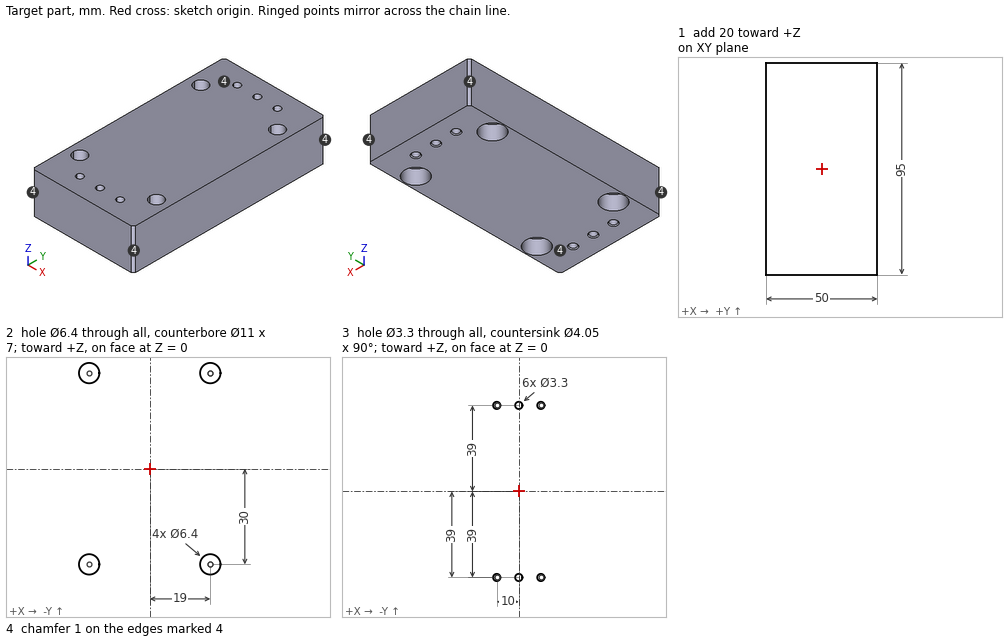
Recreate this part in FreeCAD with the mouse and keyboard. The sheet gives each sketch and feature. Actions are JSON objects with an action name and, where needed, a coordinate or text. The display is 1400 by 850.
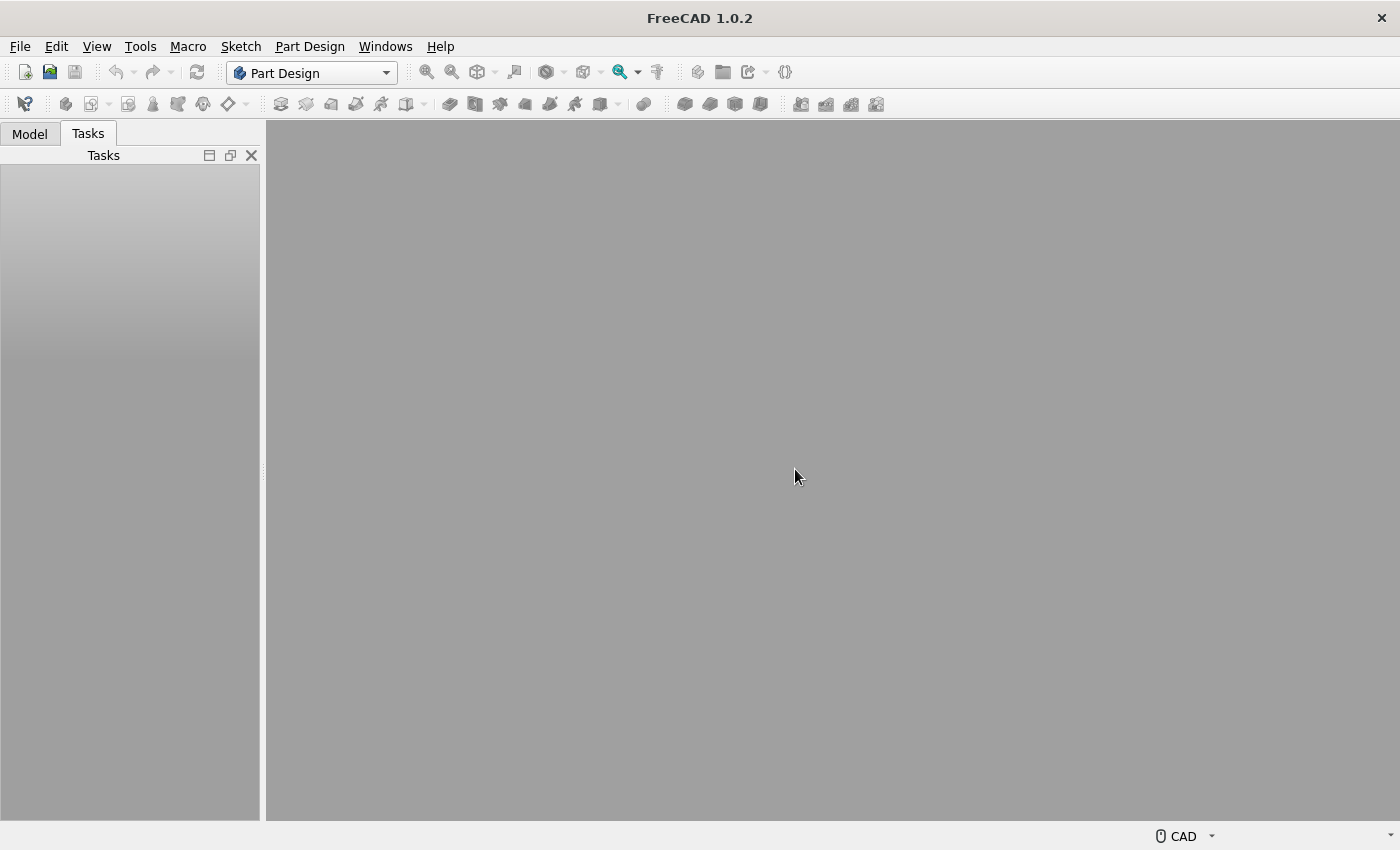
{"action": "left_click", "coordinate": [25, 72]}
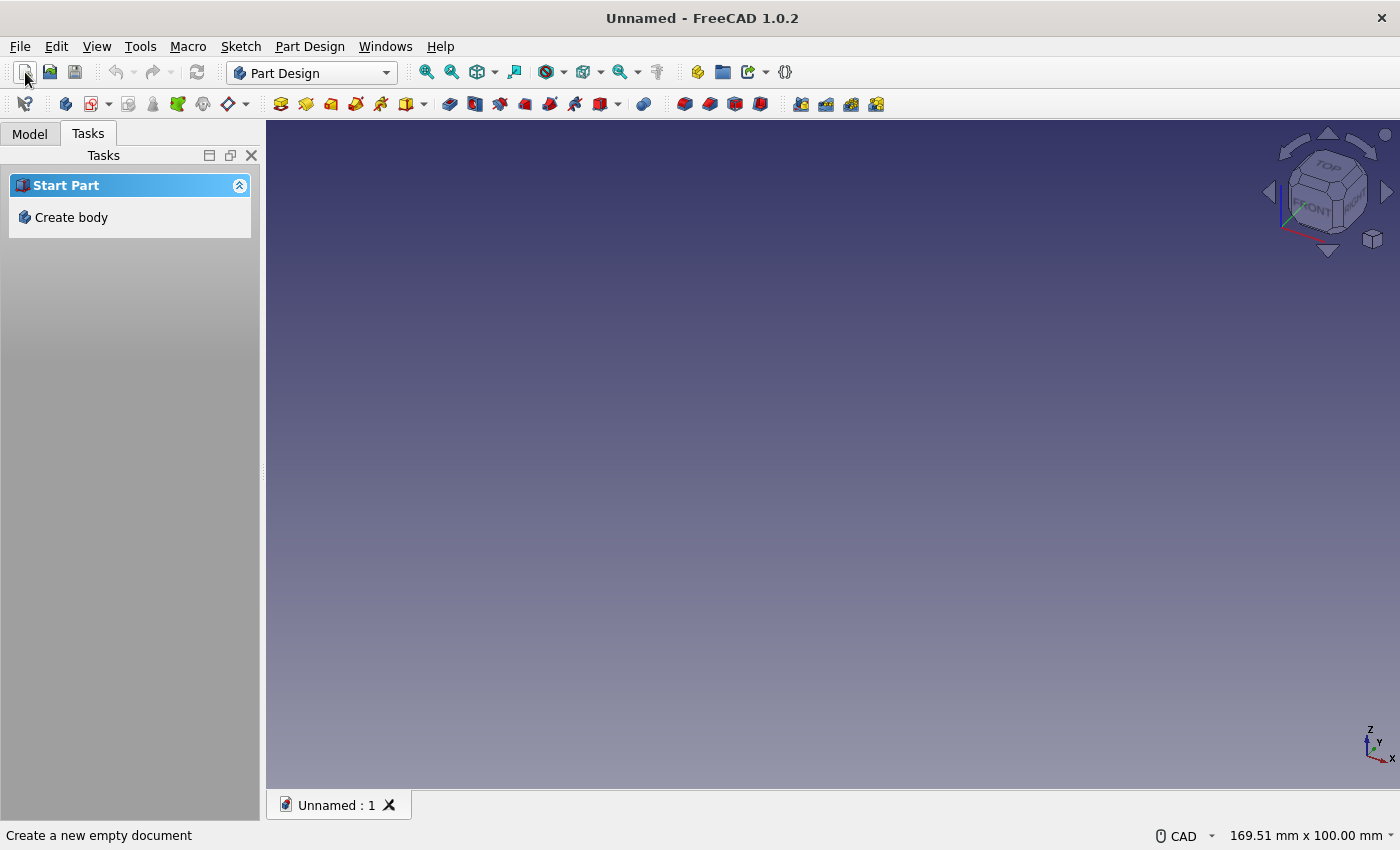
{"action": "left_click", "coordinate": [90, 104]}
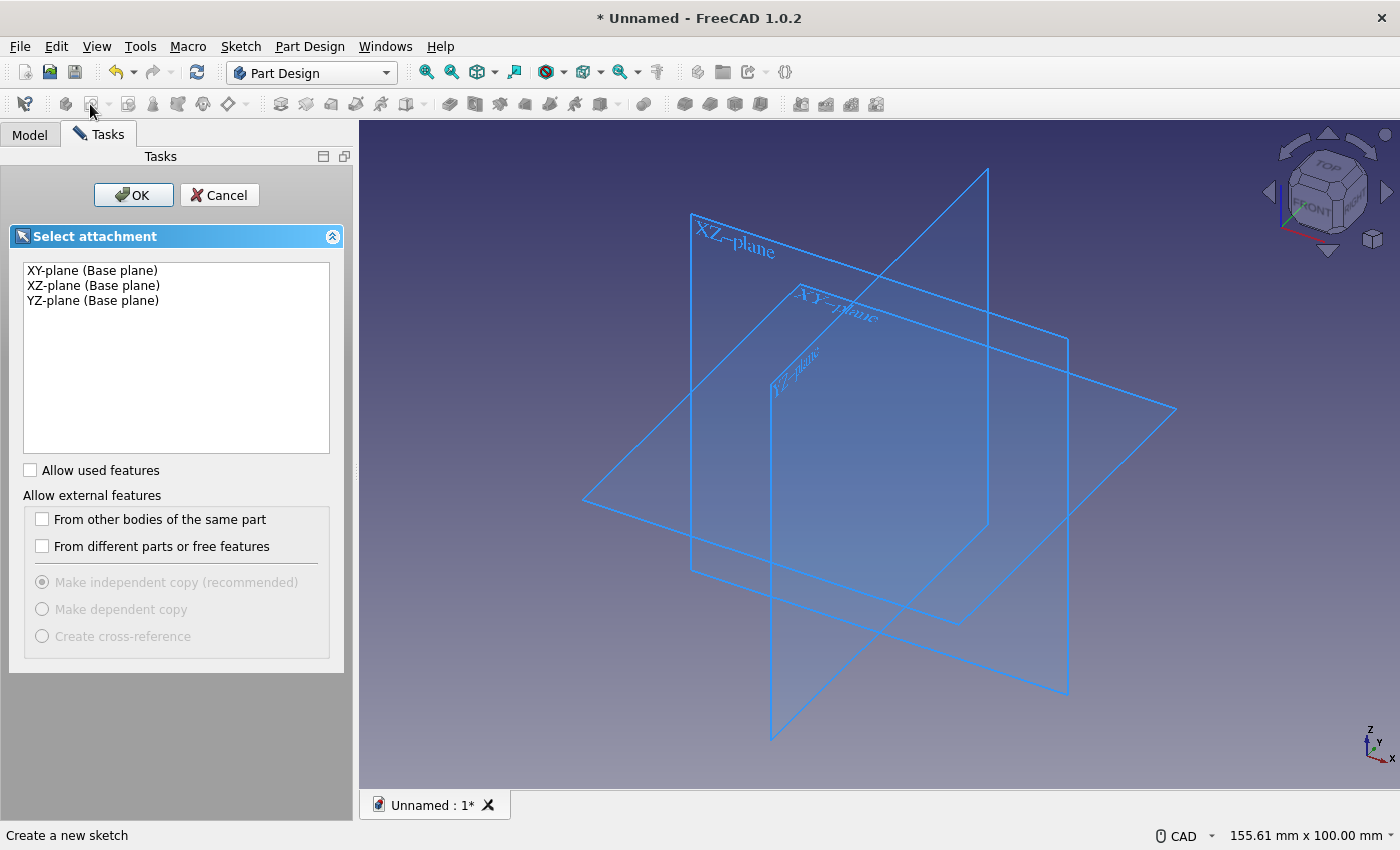
{"action": "left_click", "coordinate": [84, 270]}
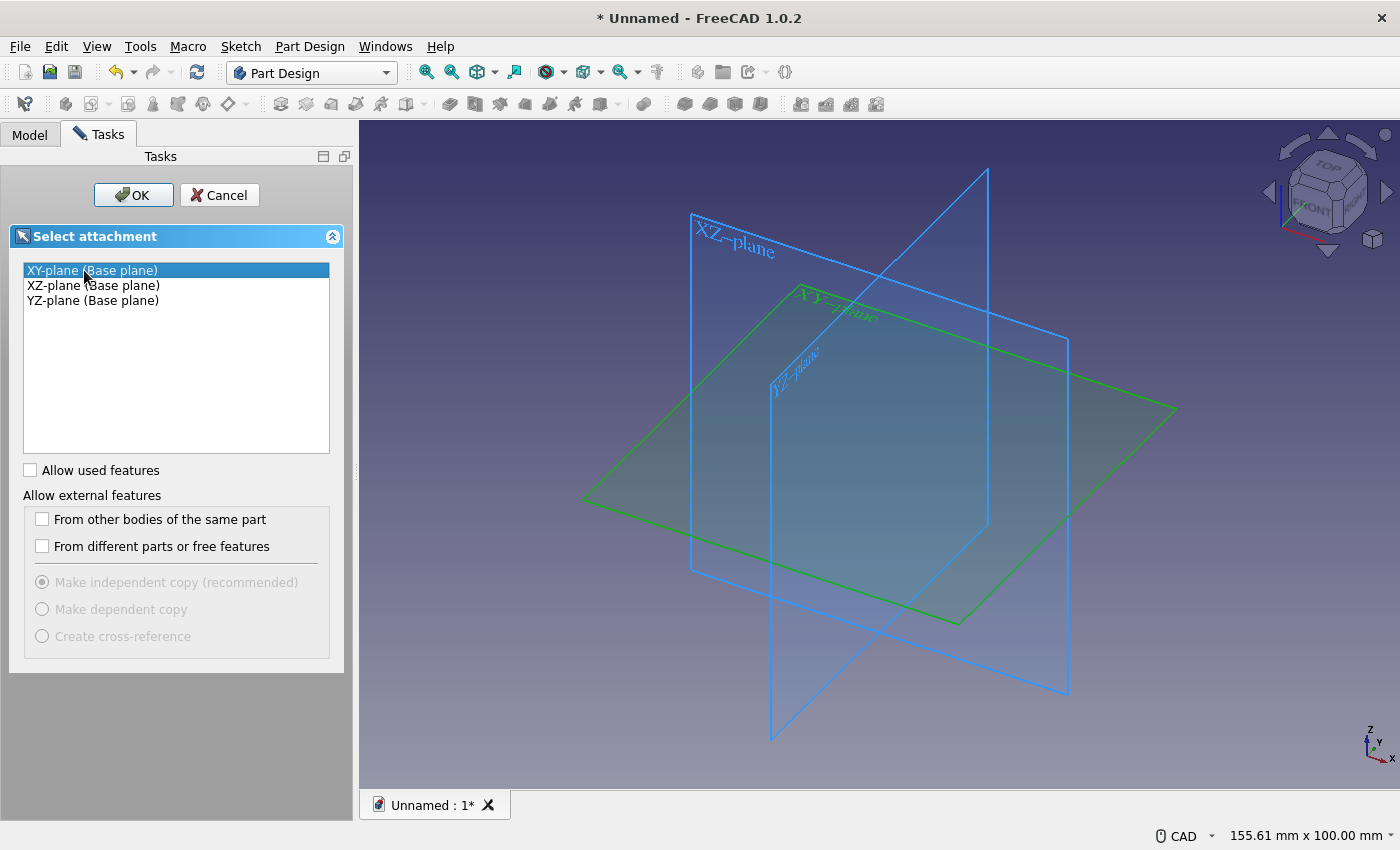
{"action": "left_click", "coordinate": [134, 195]}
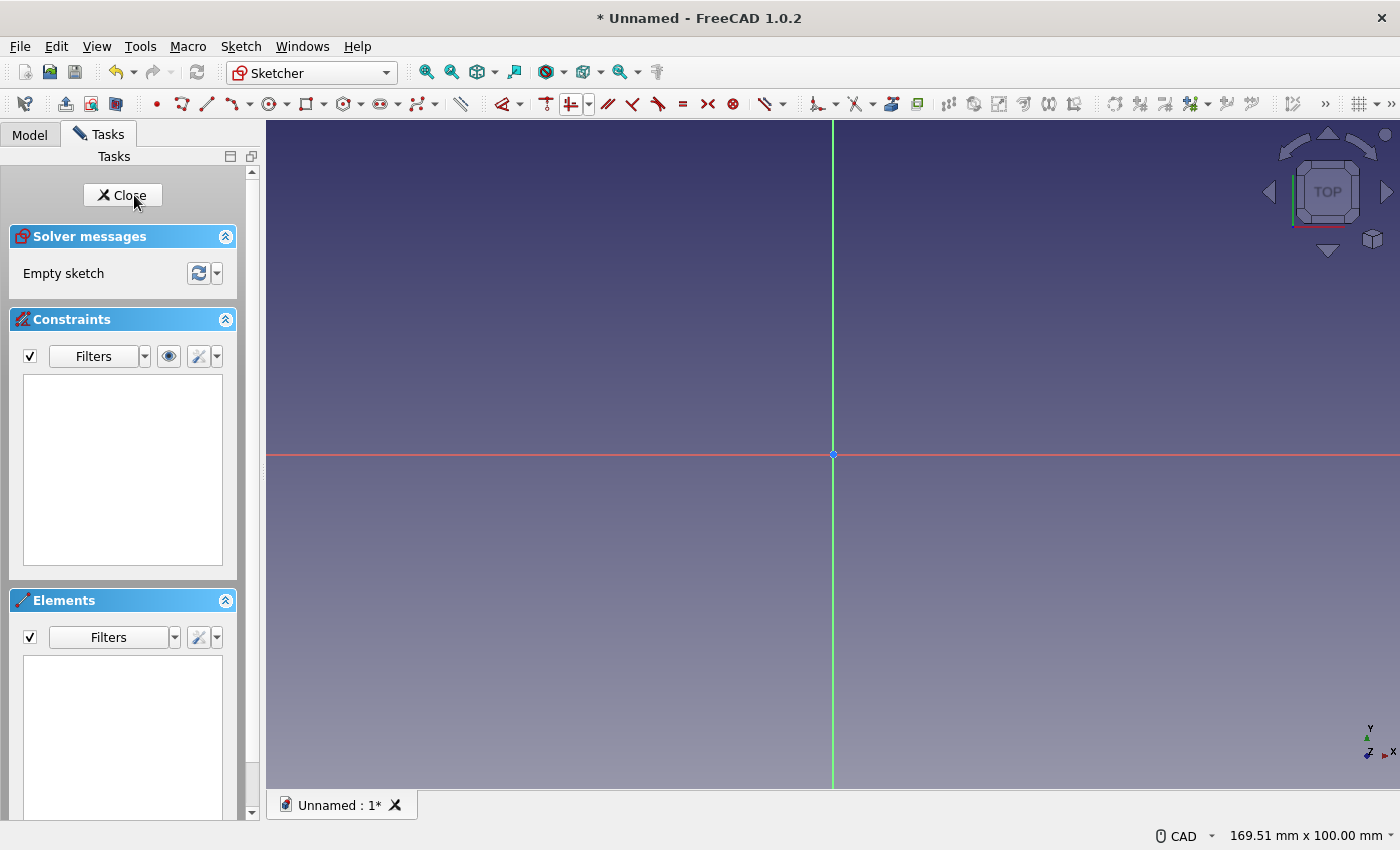
{"action": "scroll", "coordinate": [625, 455], "scroll_direction": "down", "scroll_amount": 2}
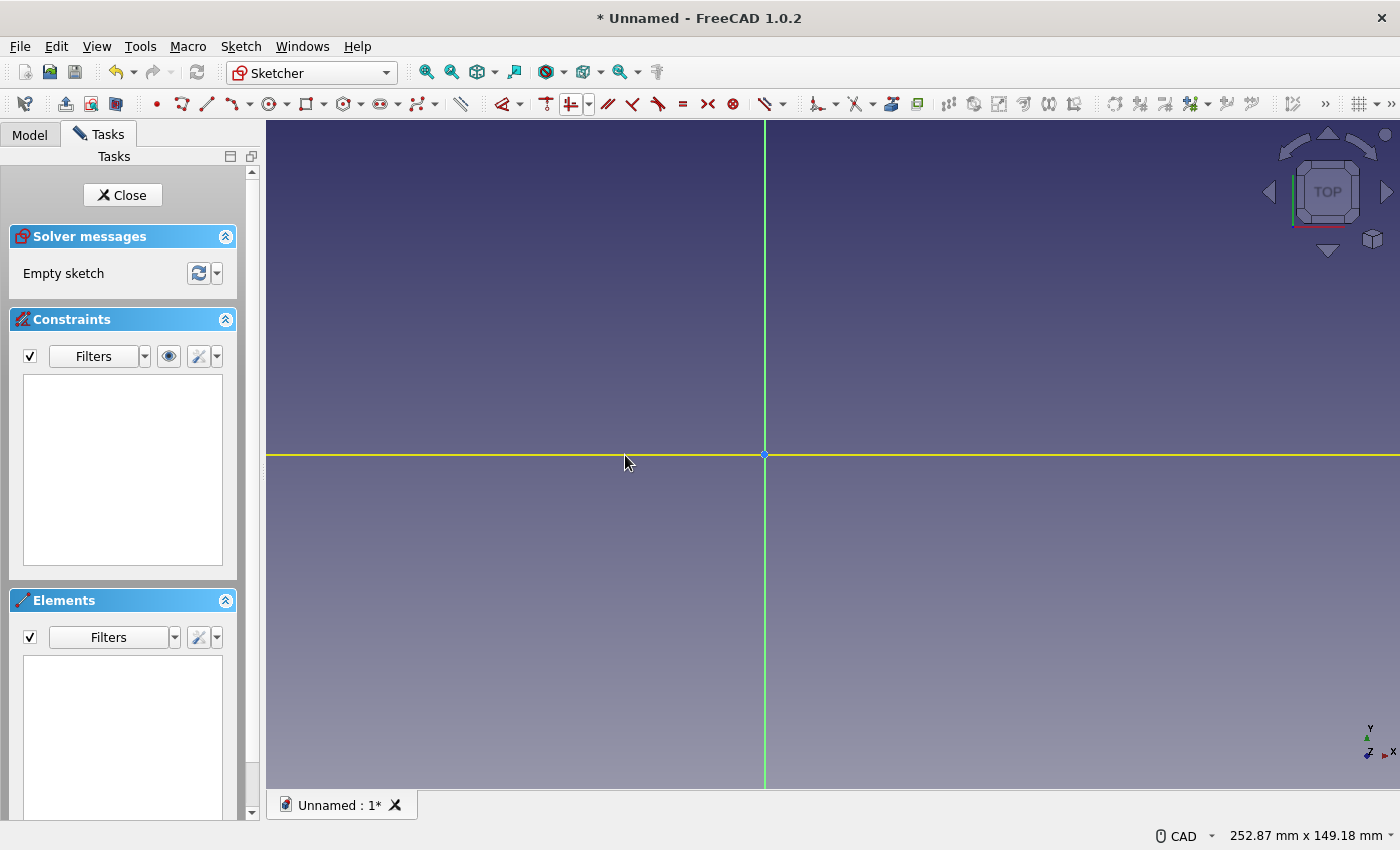
{"action": "left_click", "coordinate": [324, 104]}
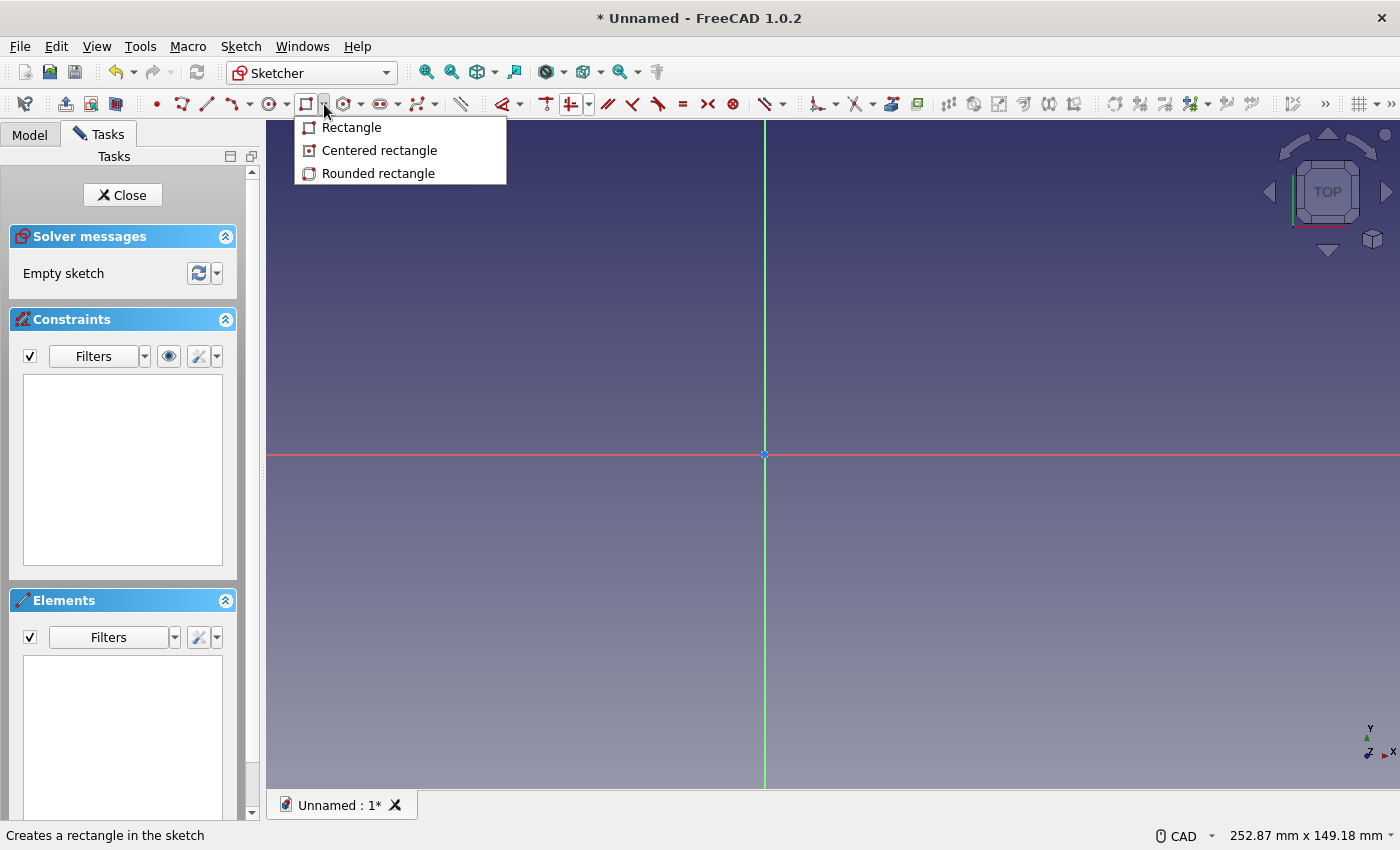
{"action": "left_click", "coordinate": [400, 150]}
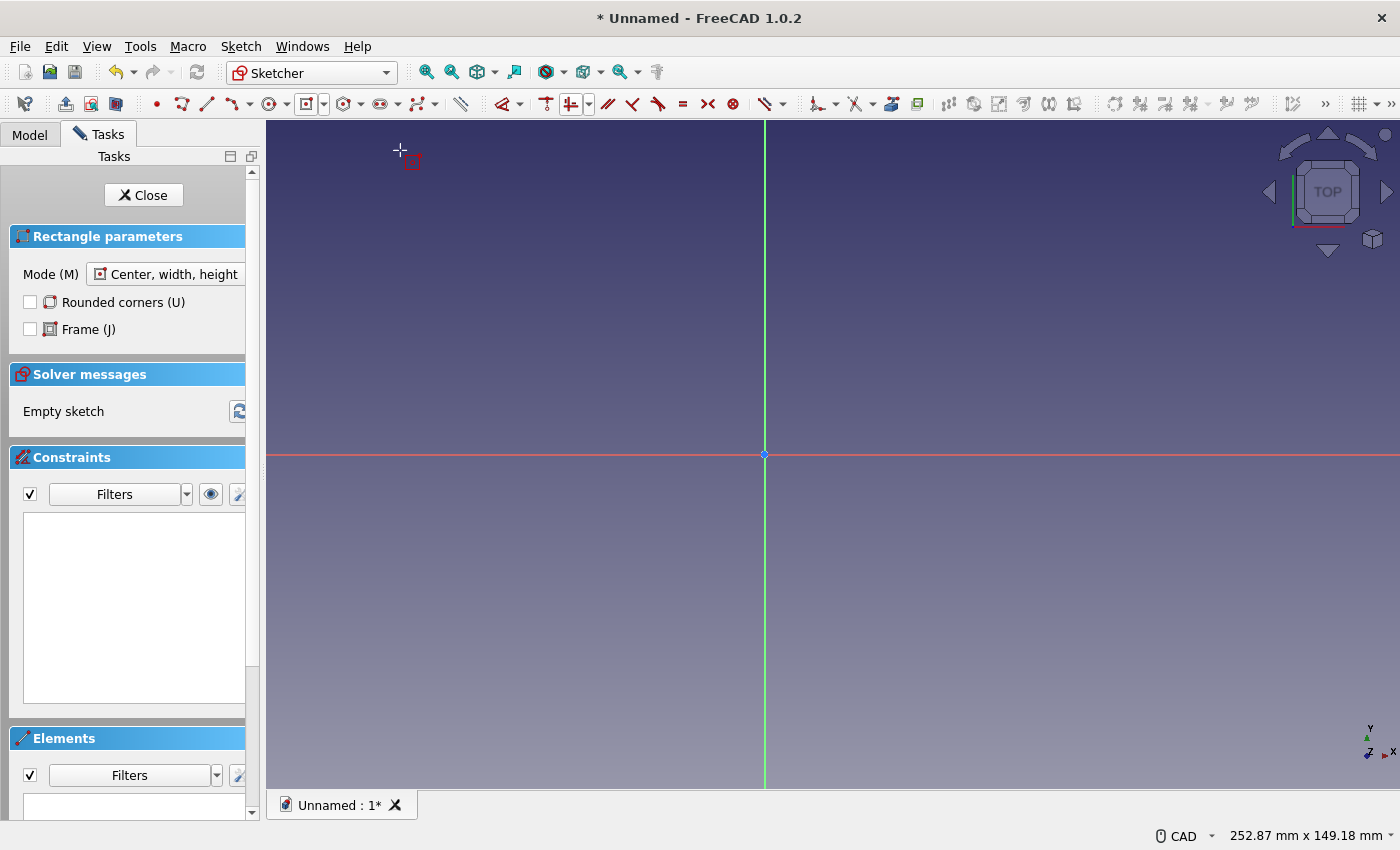
{"action": "left_click", "coordinate": [765, 455]}
{"action": "left_click", "coordinate": [877, 242]}
{"action": "key", "text": "Escape"}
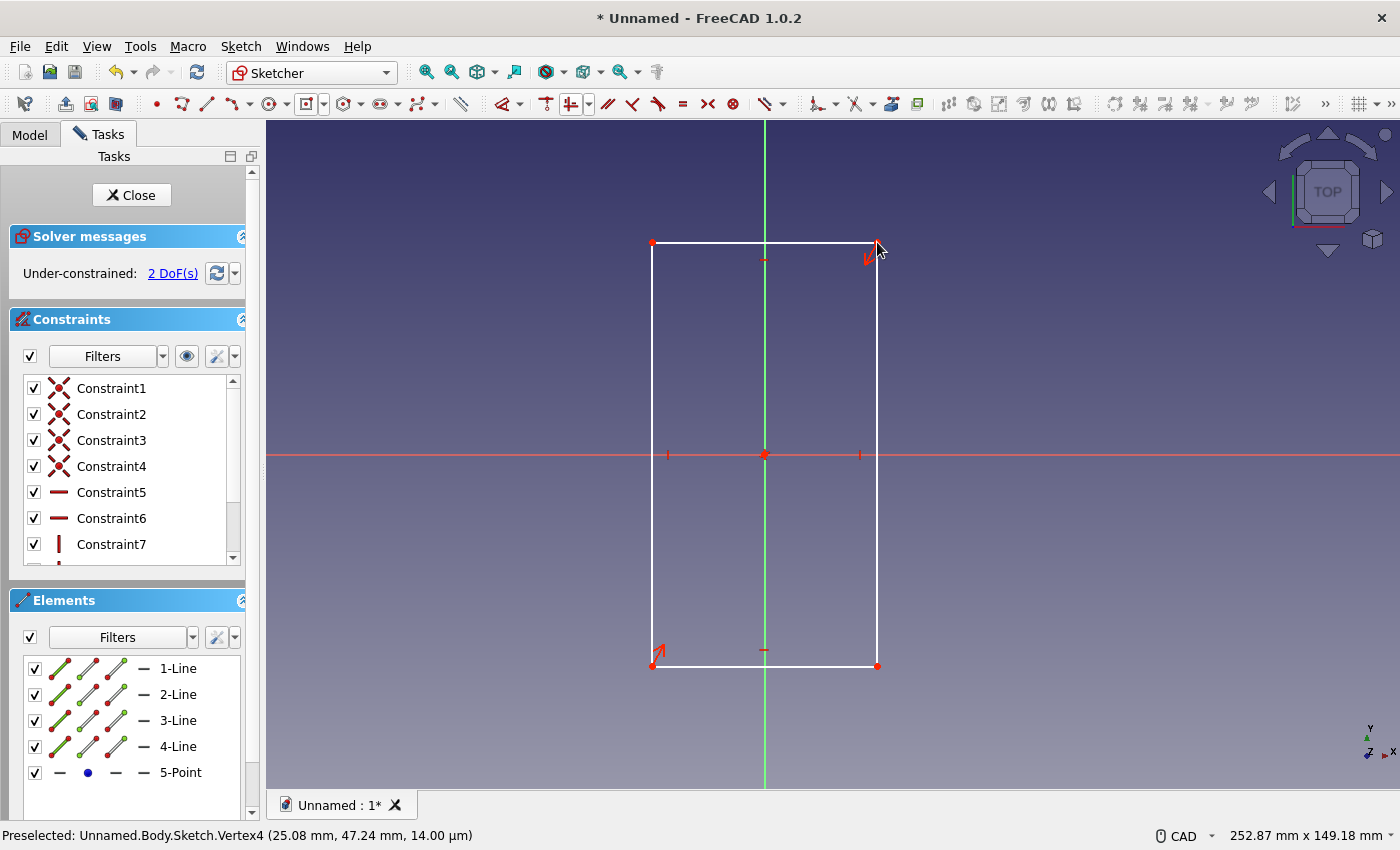
{"action": "left_click", "coordinate": [502, 104]}